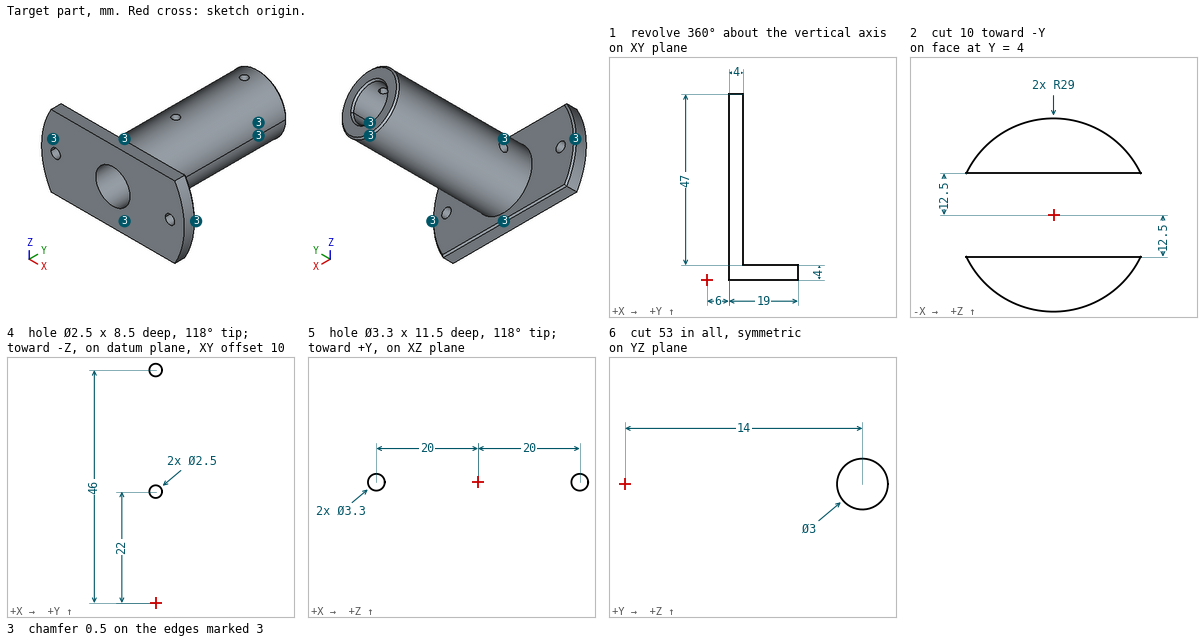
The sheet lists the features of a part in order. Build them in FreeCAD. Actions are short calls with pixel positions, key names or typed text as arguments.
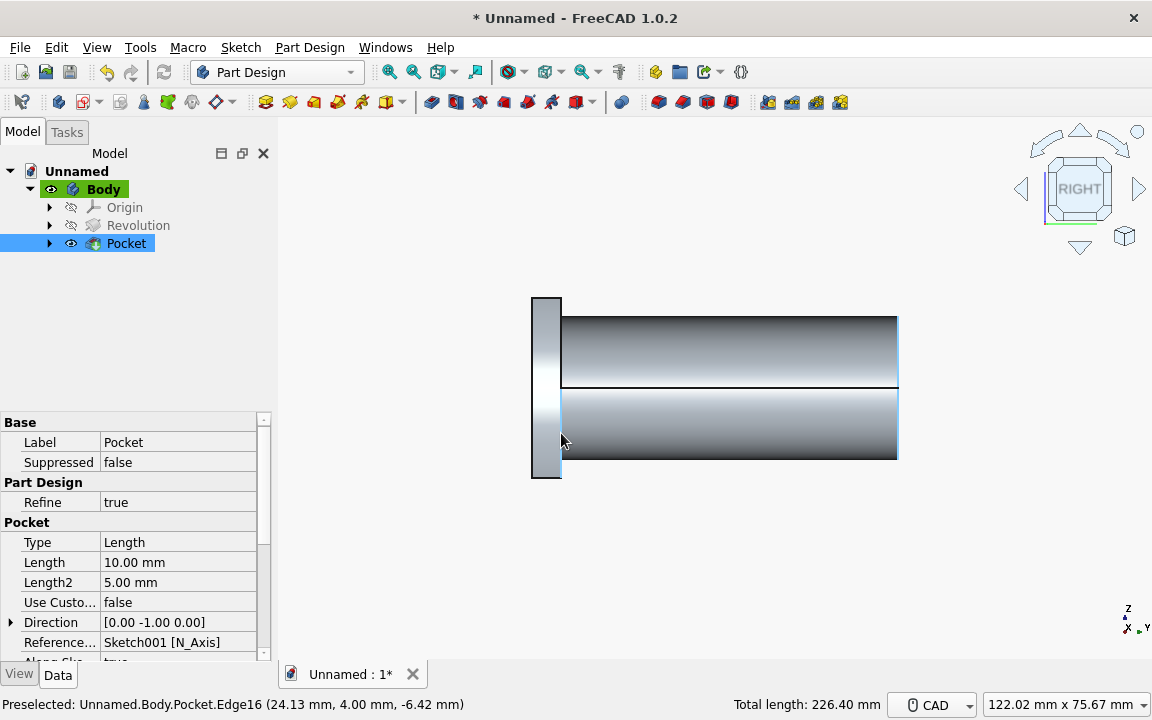
click(684, 102)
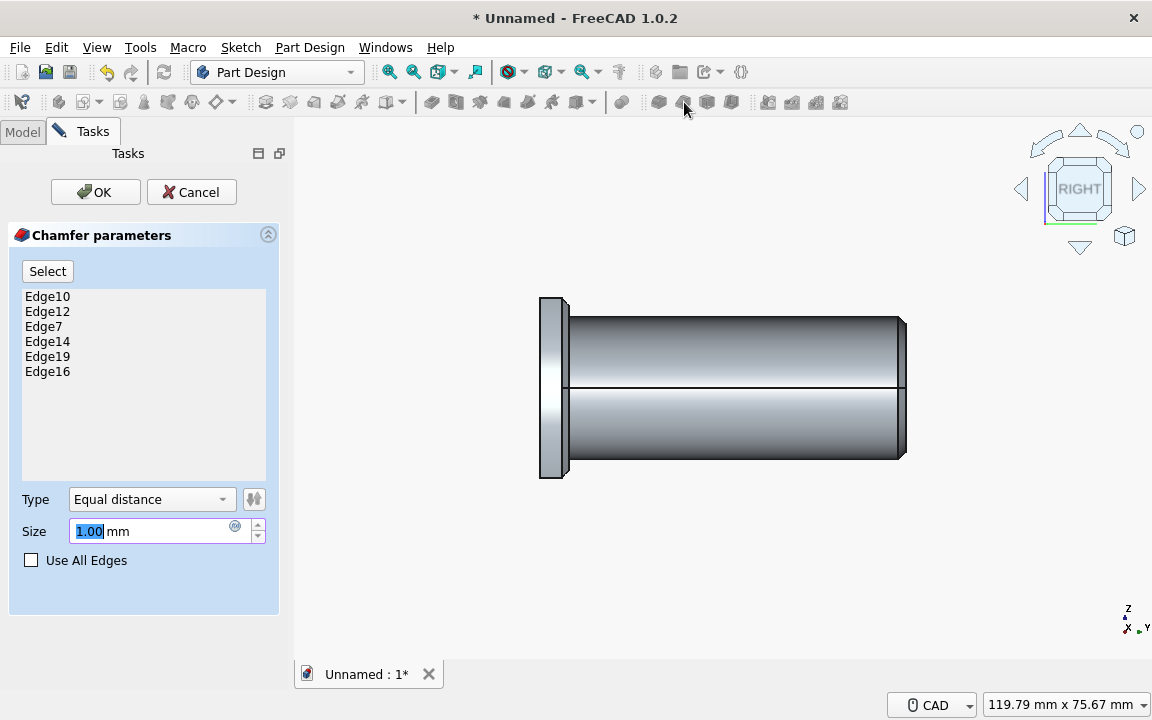
text(0.5)
key(Tab)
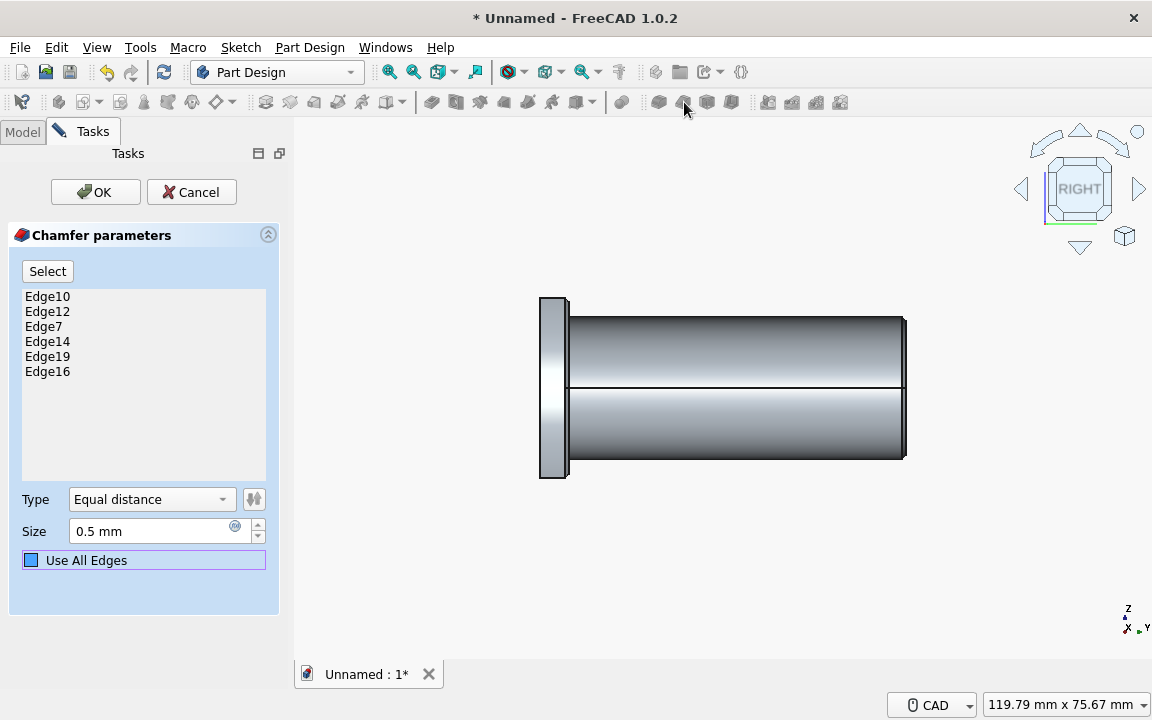
click(96, 192)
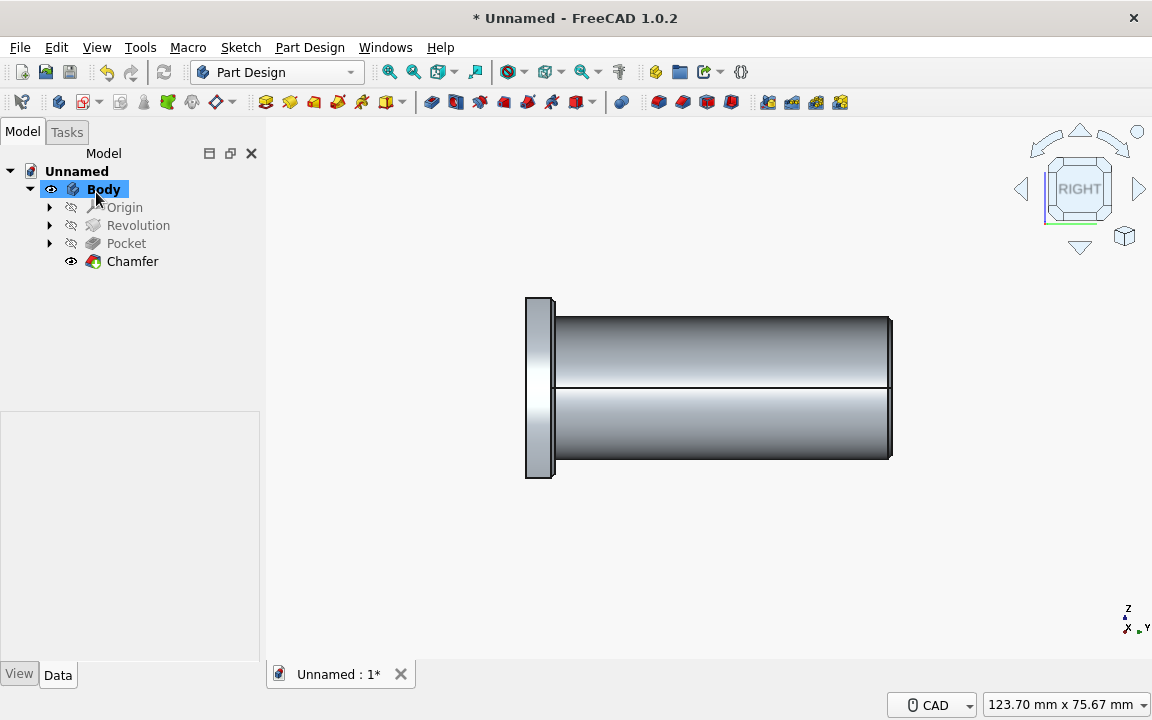
key(v)
key(f)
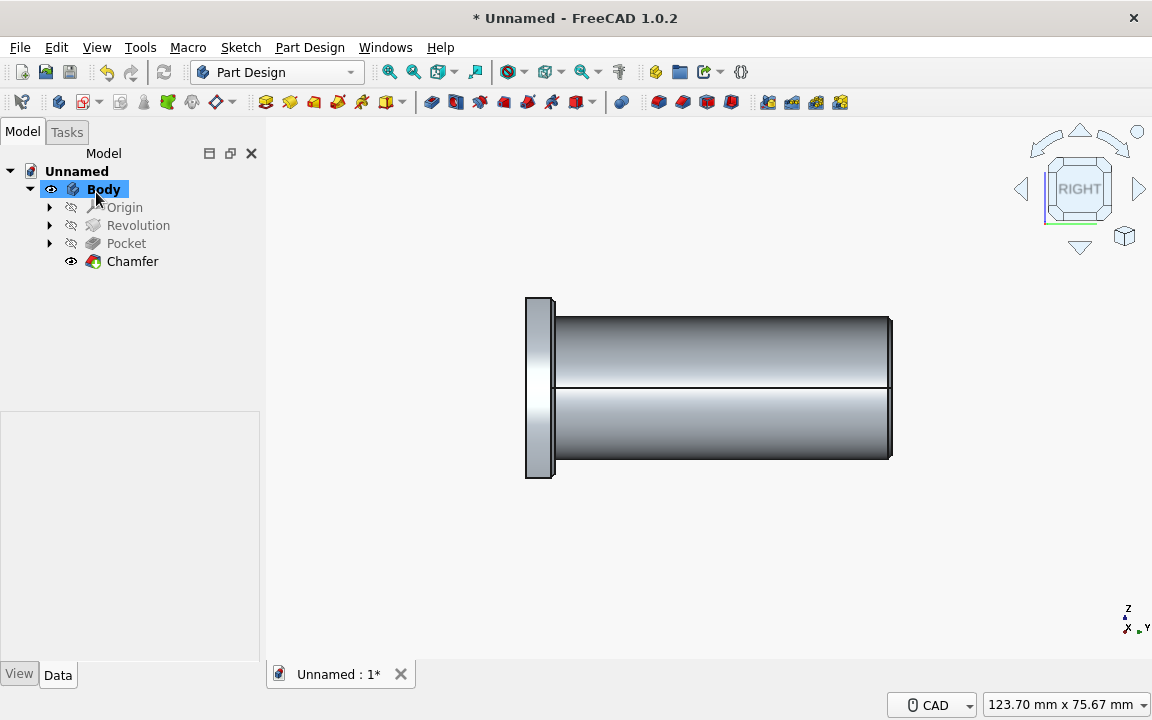
click(50, 207)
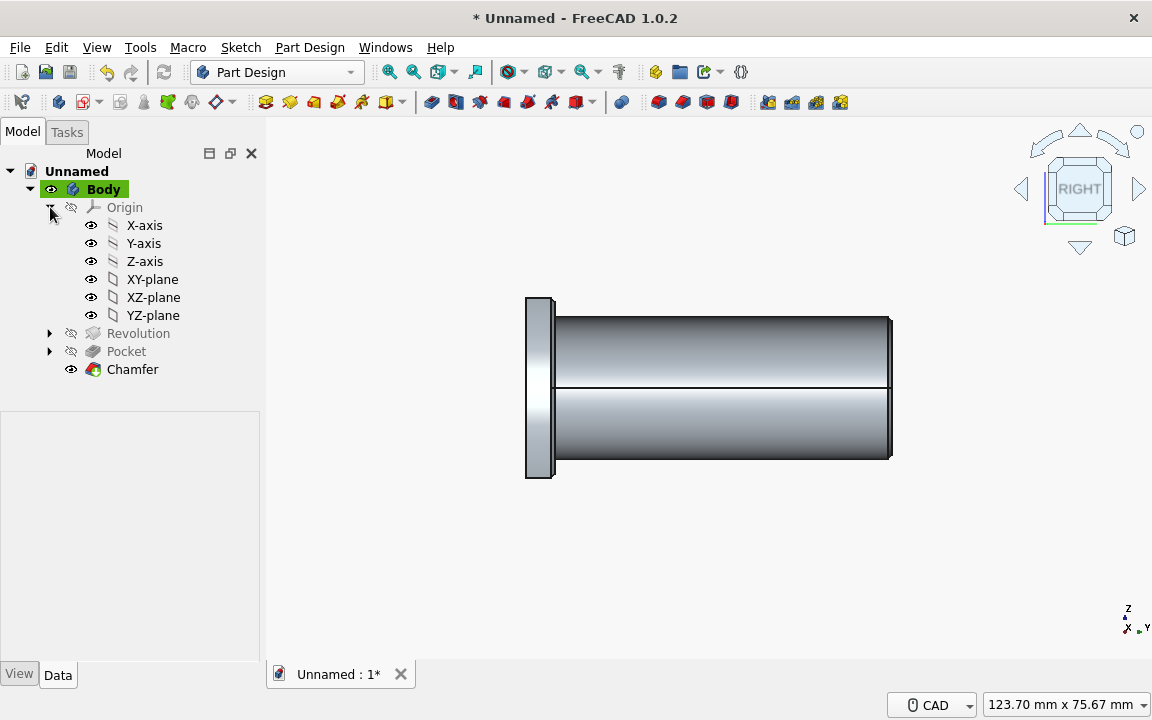
click(136, 279)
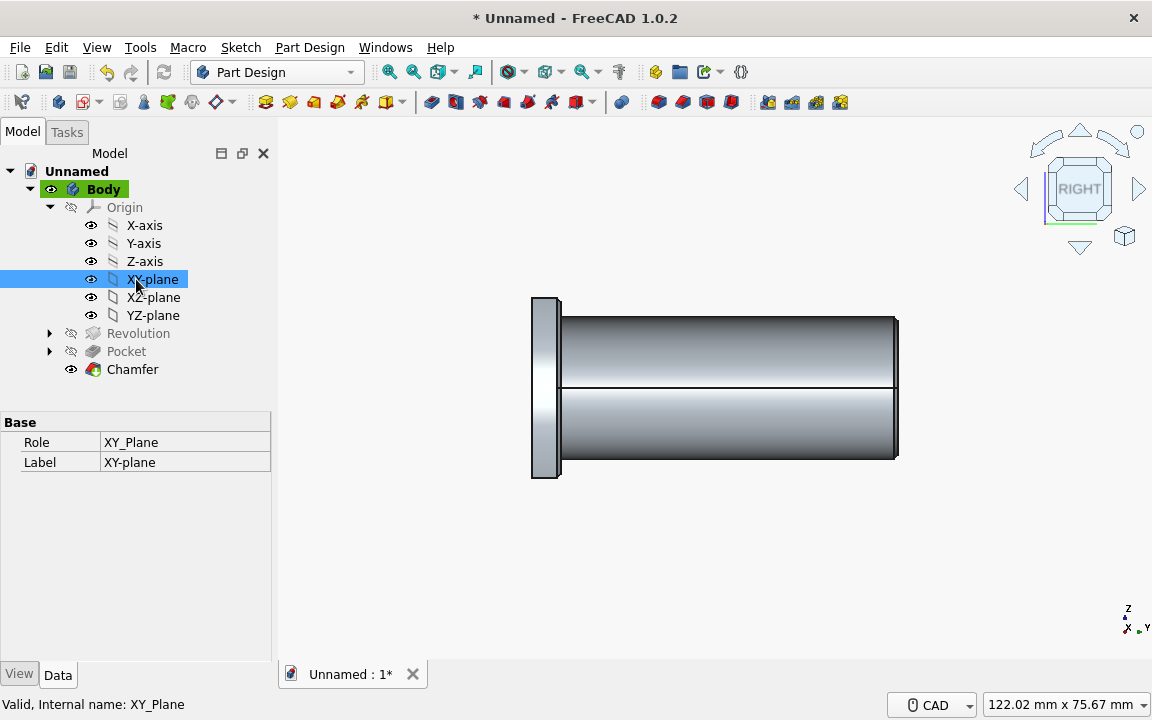
click(216, 102)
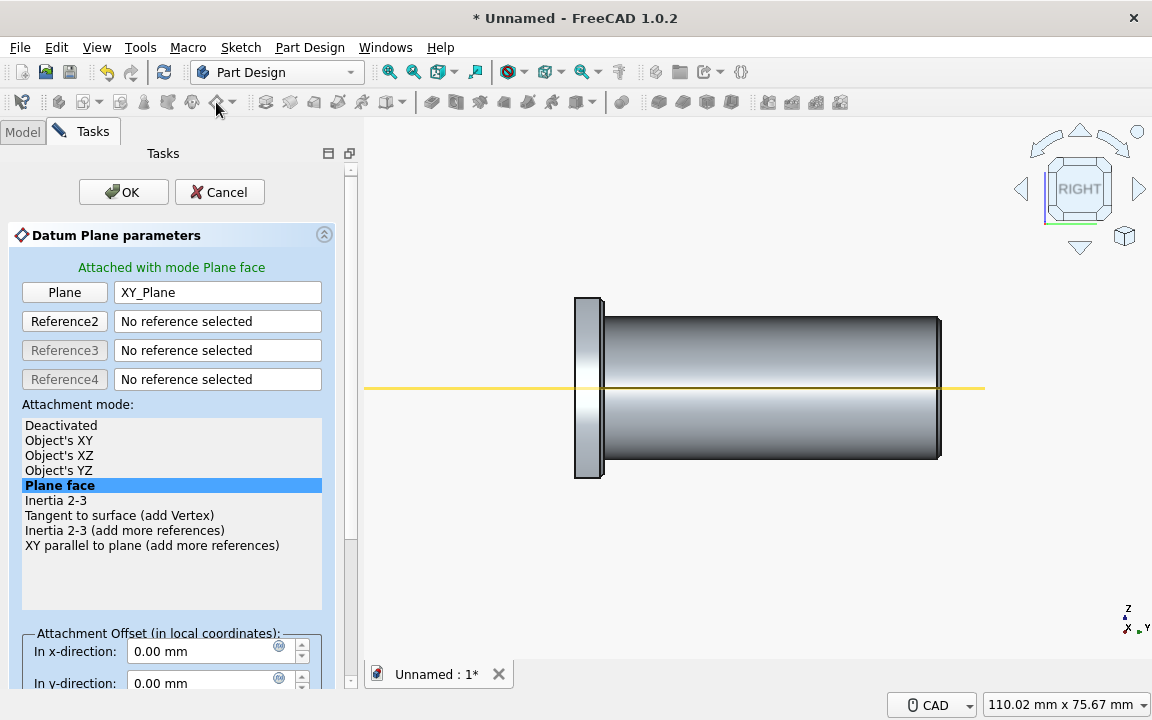
scroll(351, 426, down, 2)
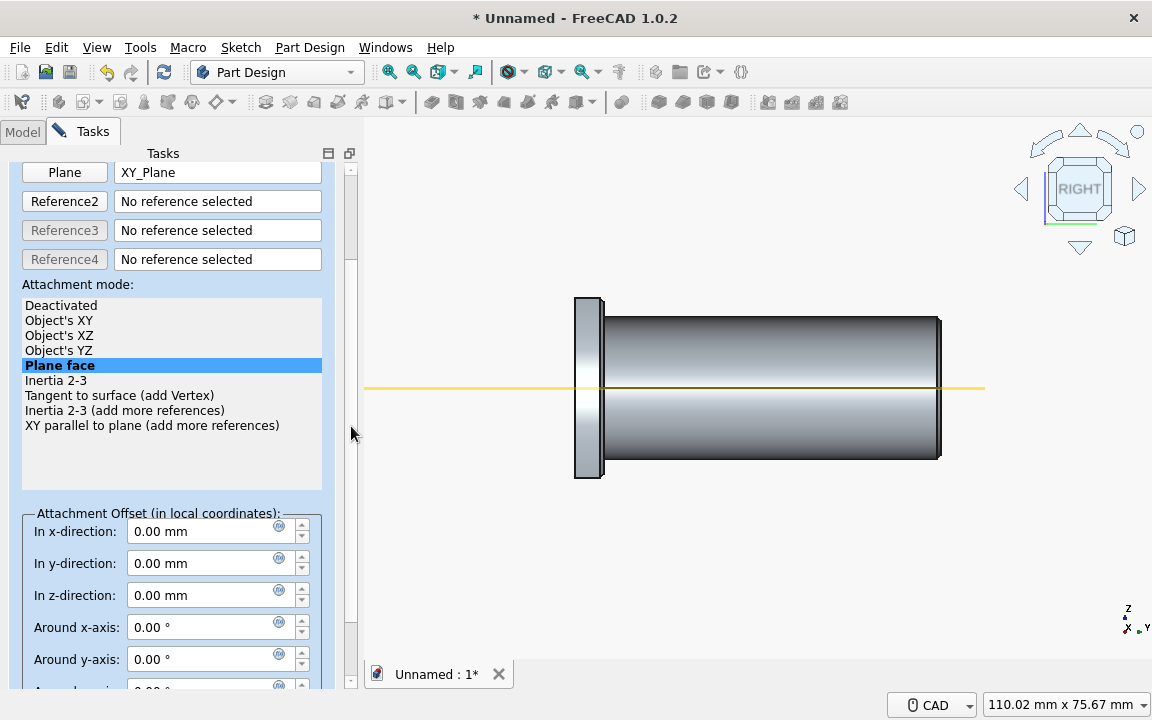
triple_click(210, 595)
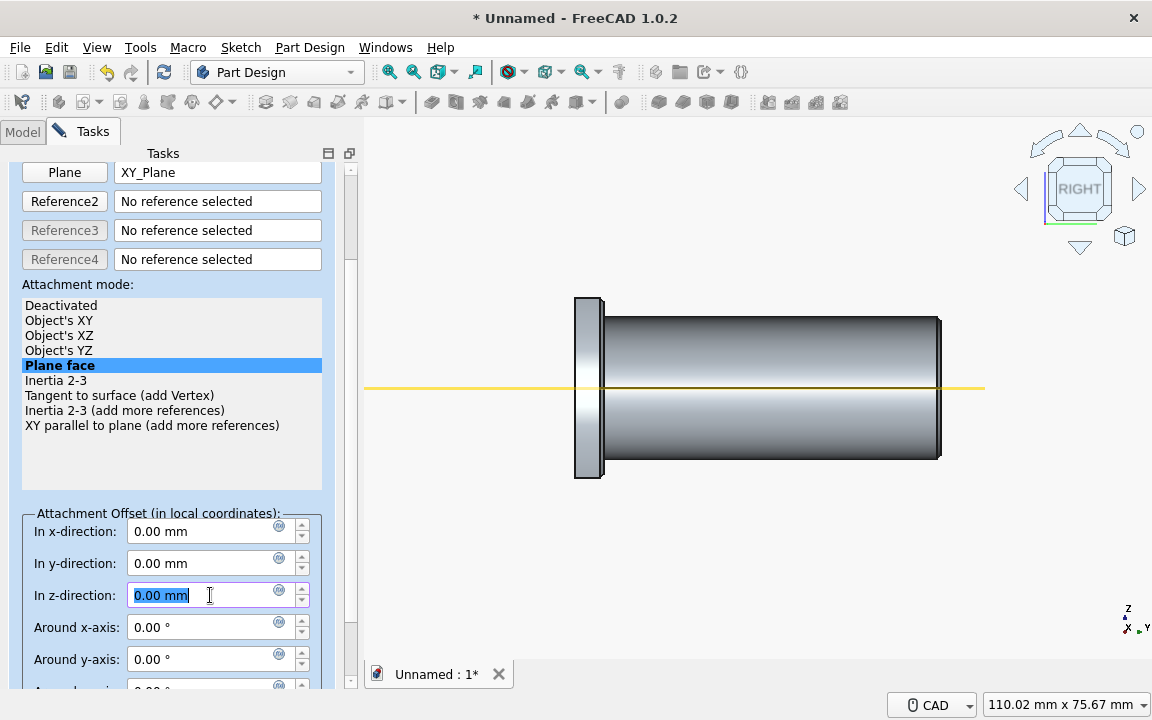
text(10)
key(Tab)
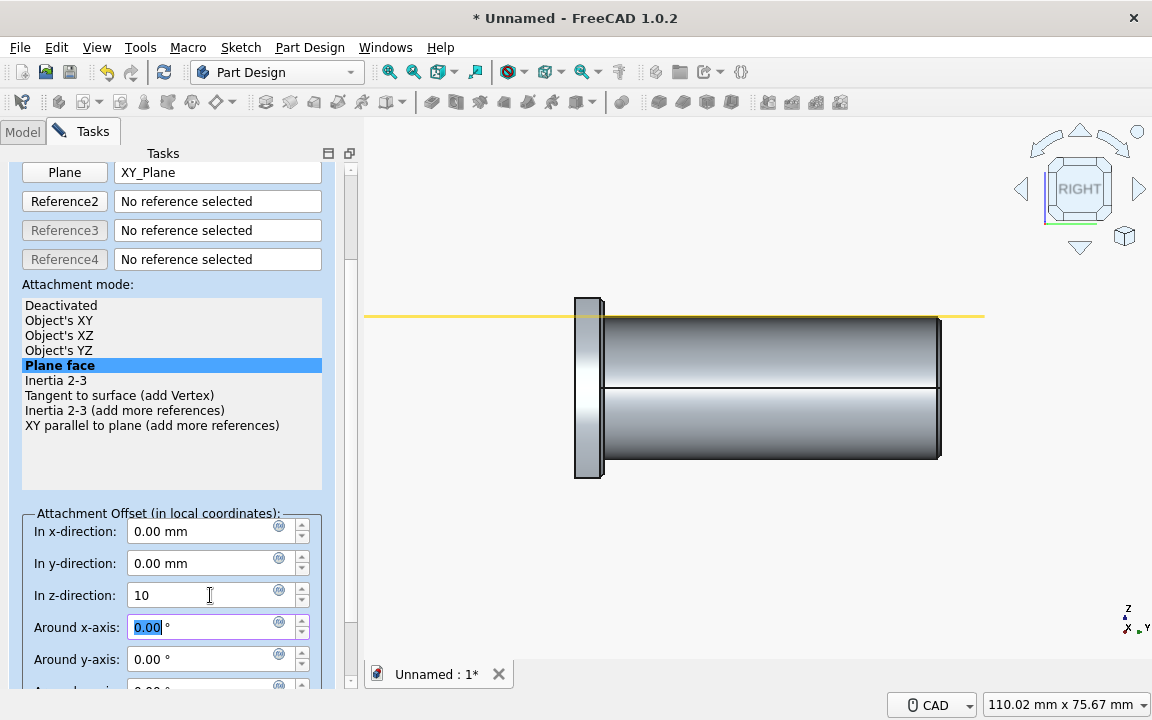
scroll(351, 426, up, 3)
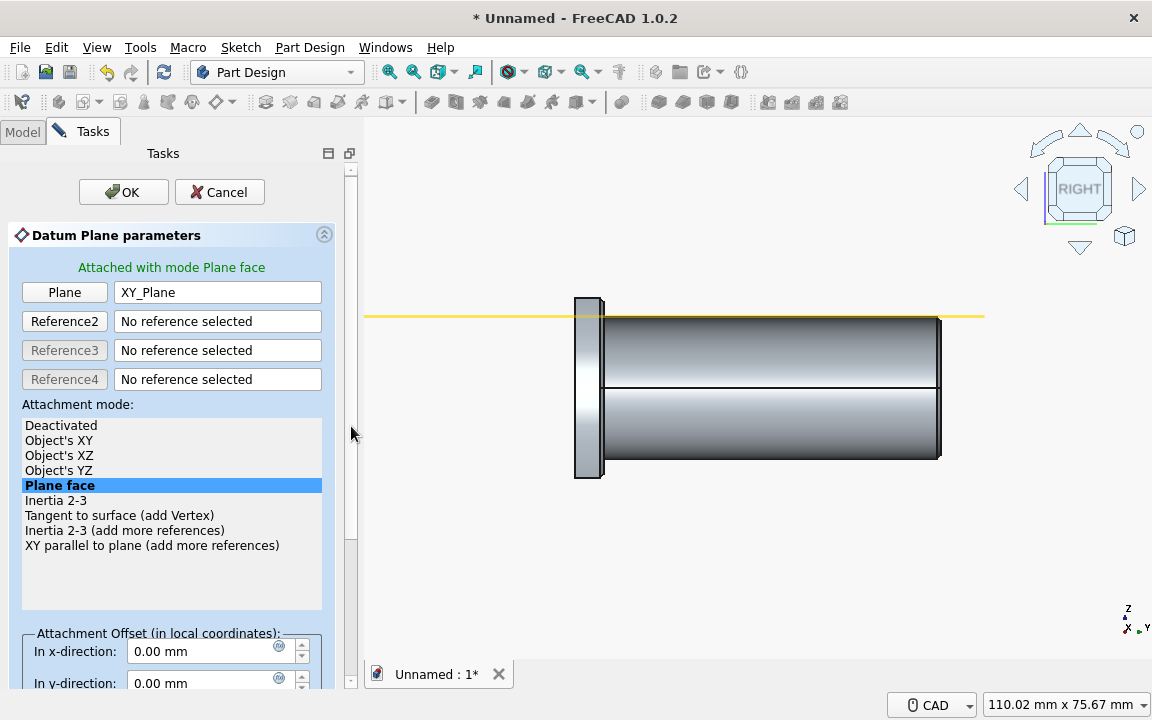
click(124, 192)